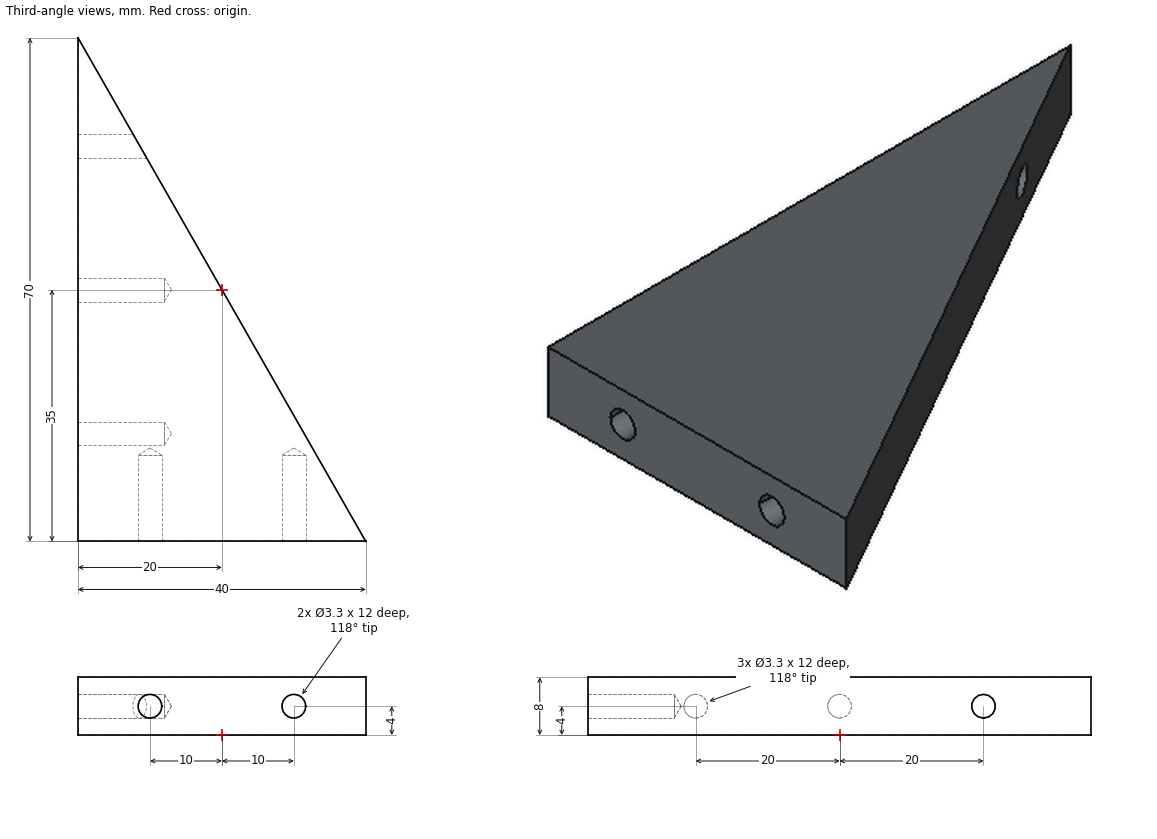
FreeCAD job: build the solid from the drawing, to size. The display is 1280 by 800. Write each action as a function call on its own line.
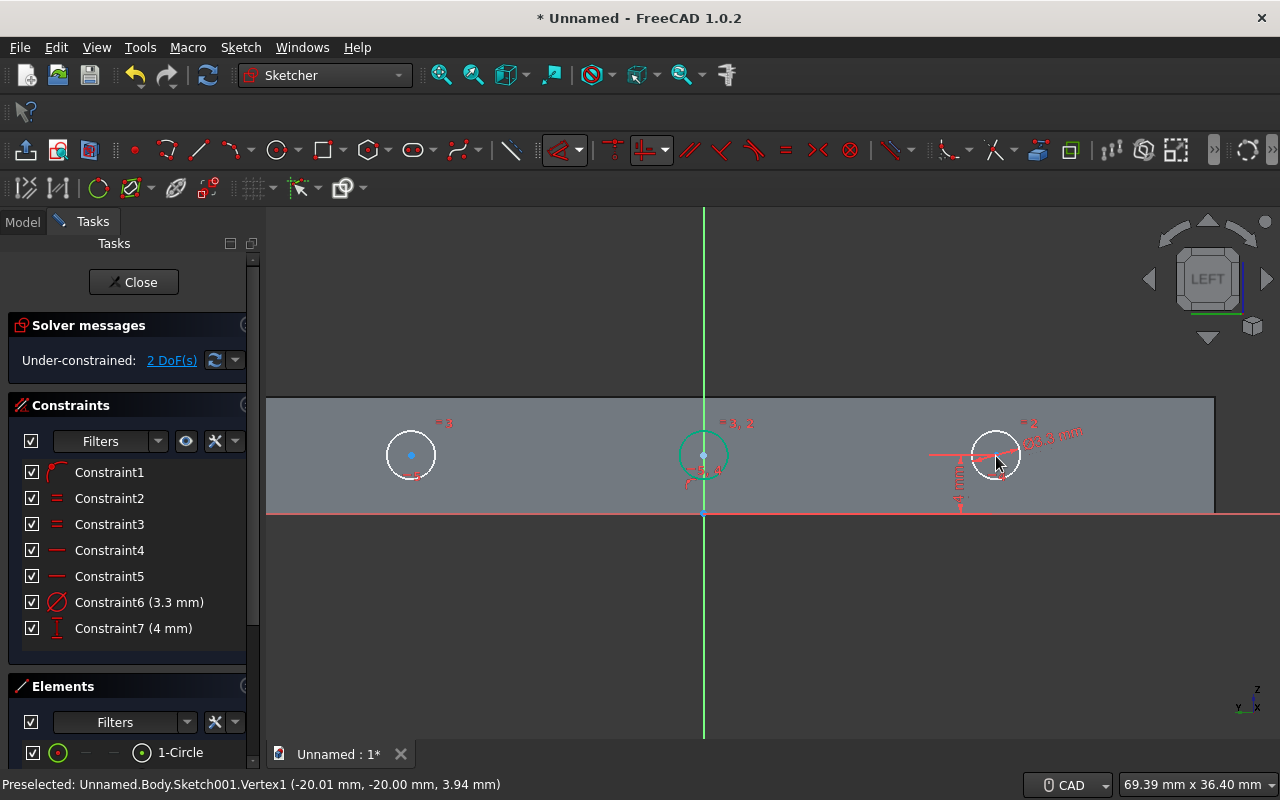
click(996, 455)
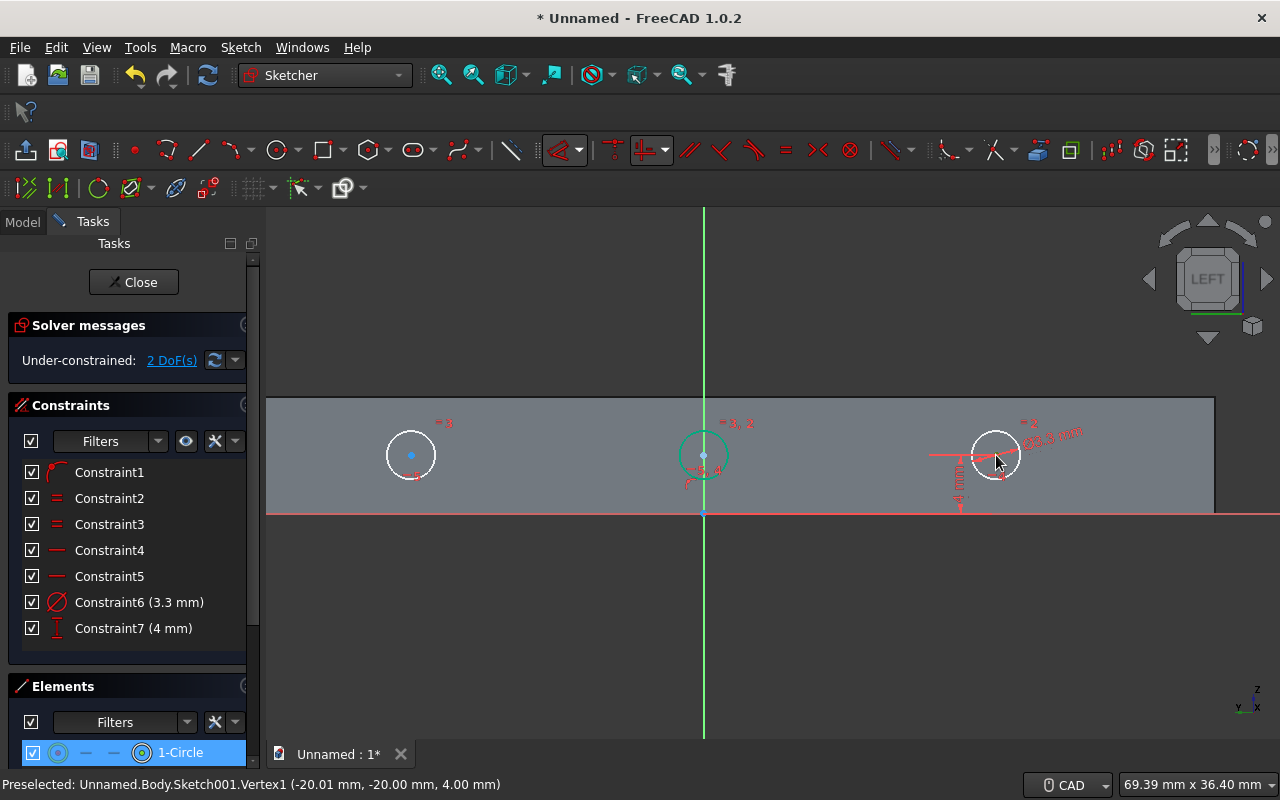
click(582, 150)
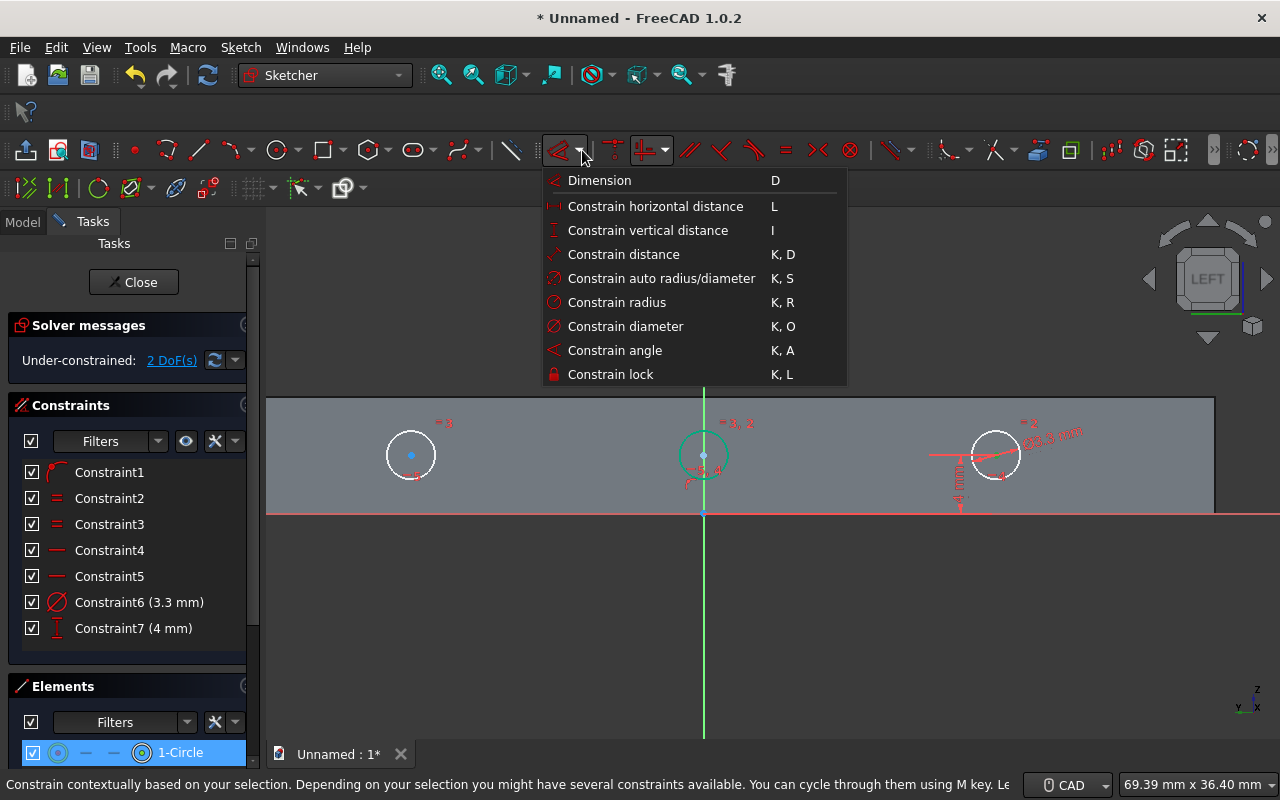
click(695, 206)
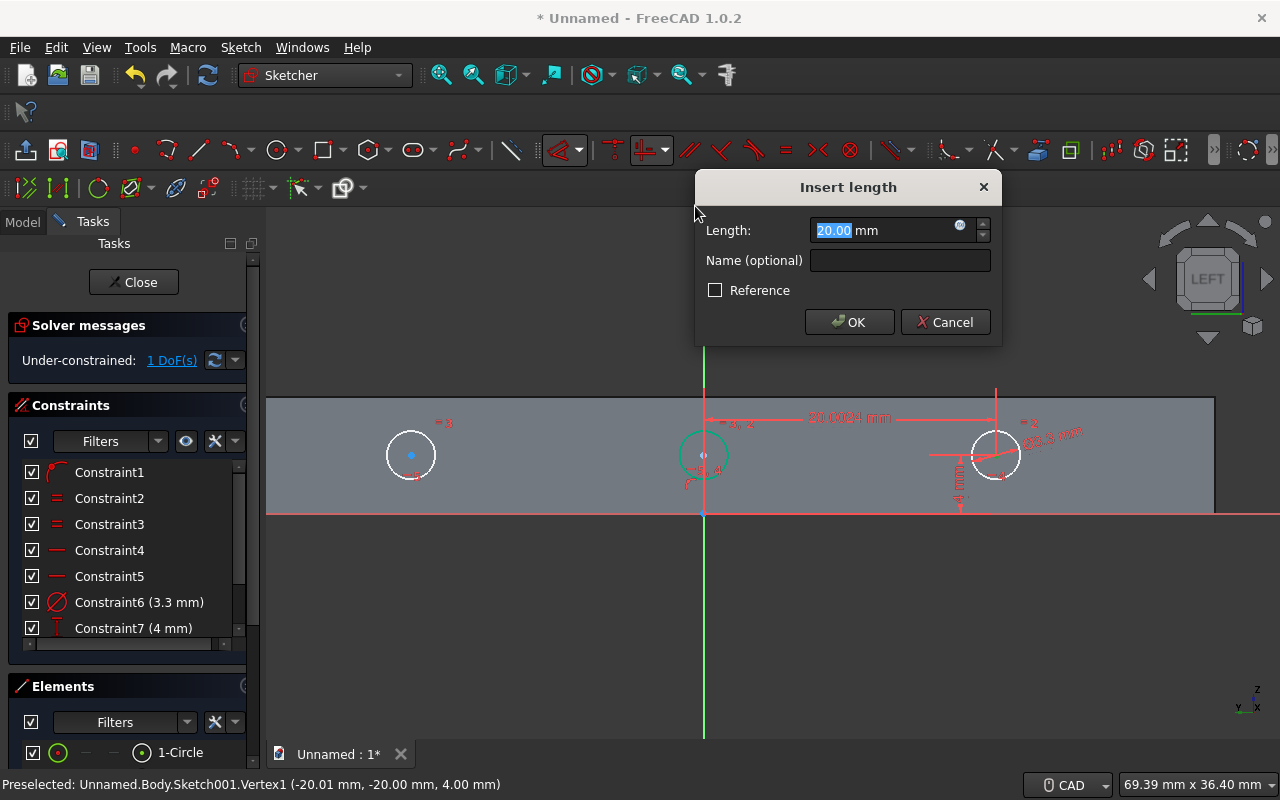
text(20)
key(Return)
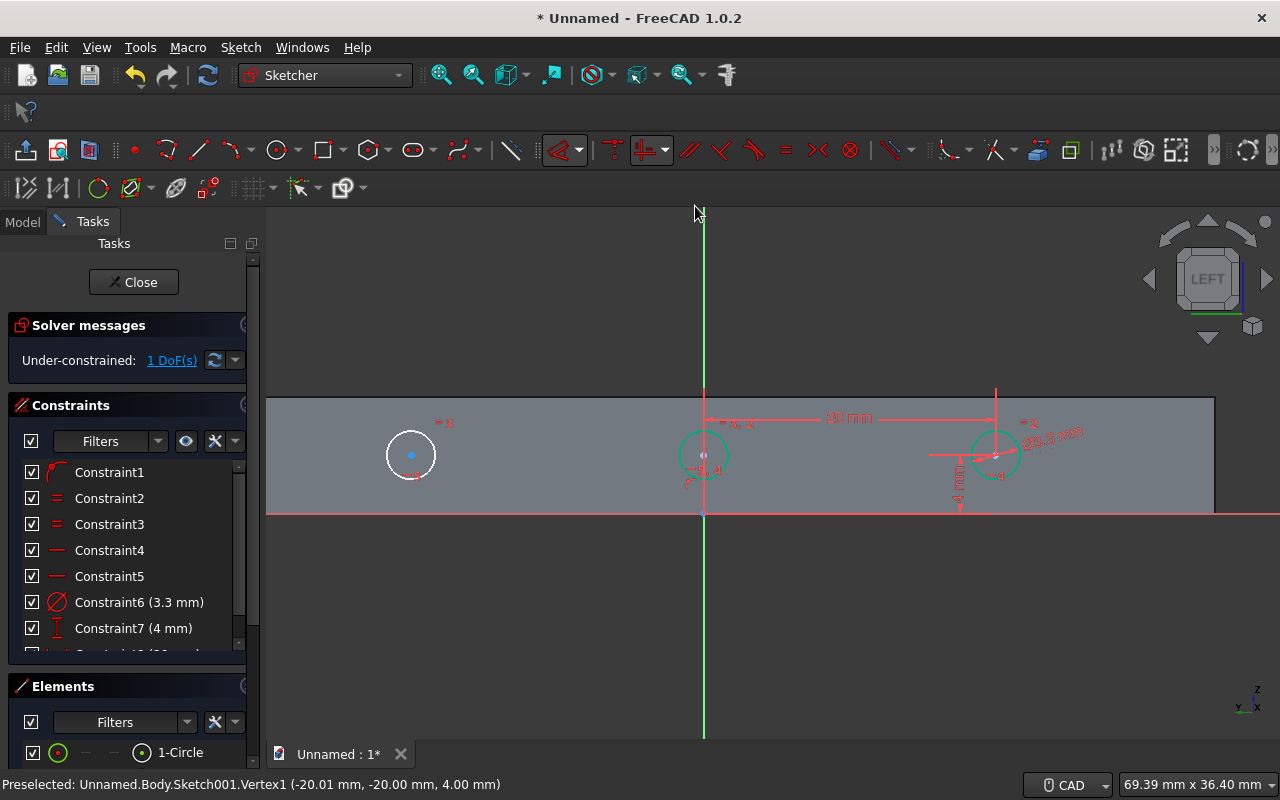
click(411, 455)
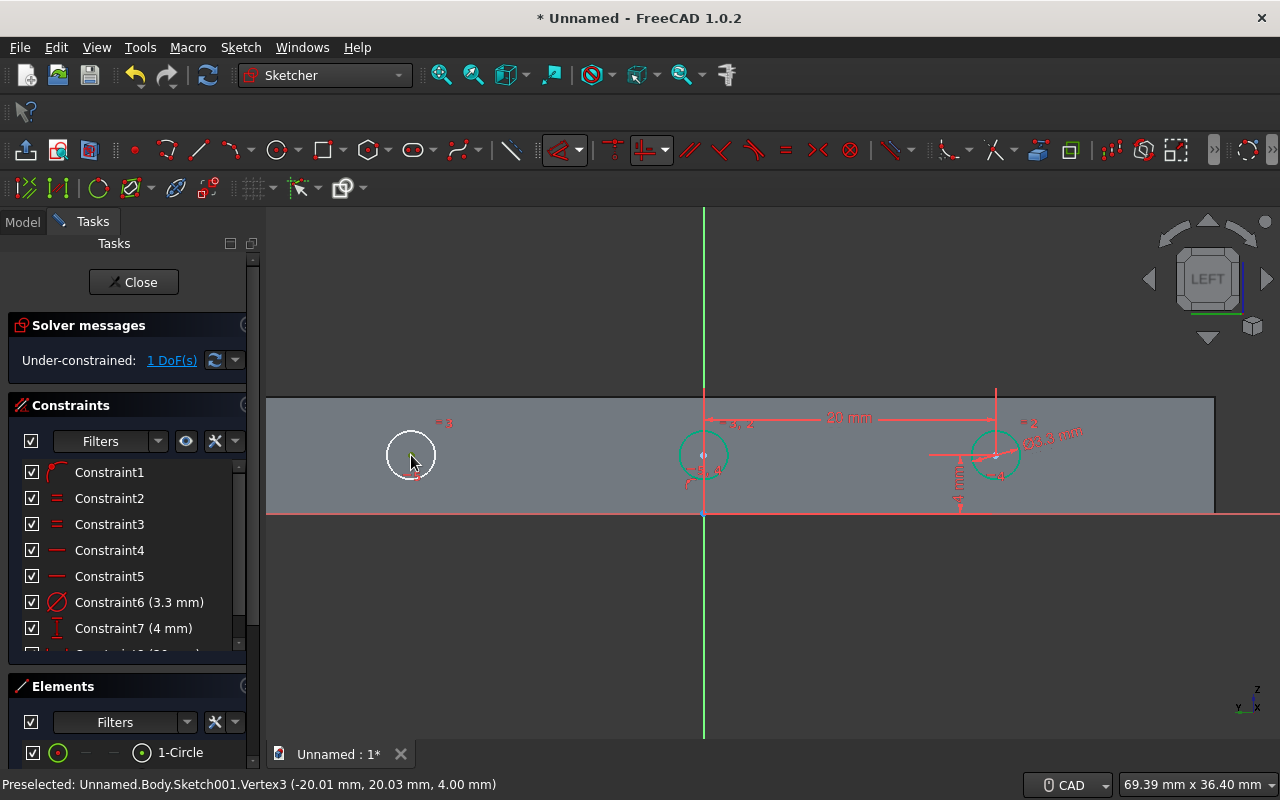
key(l)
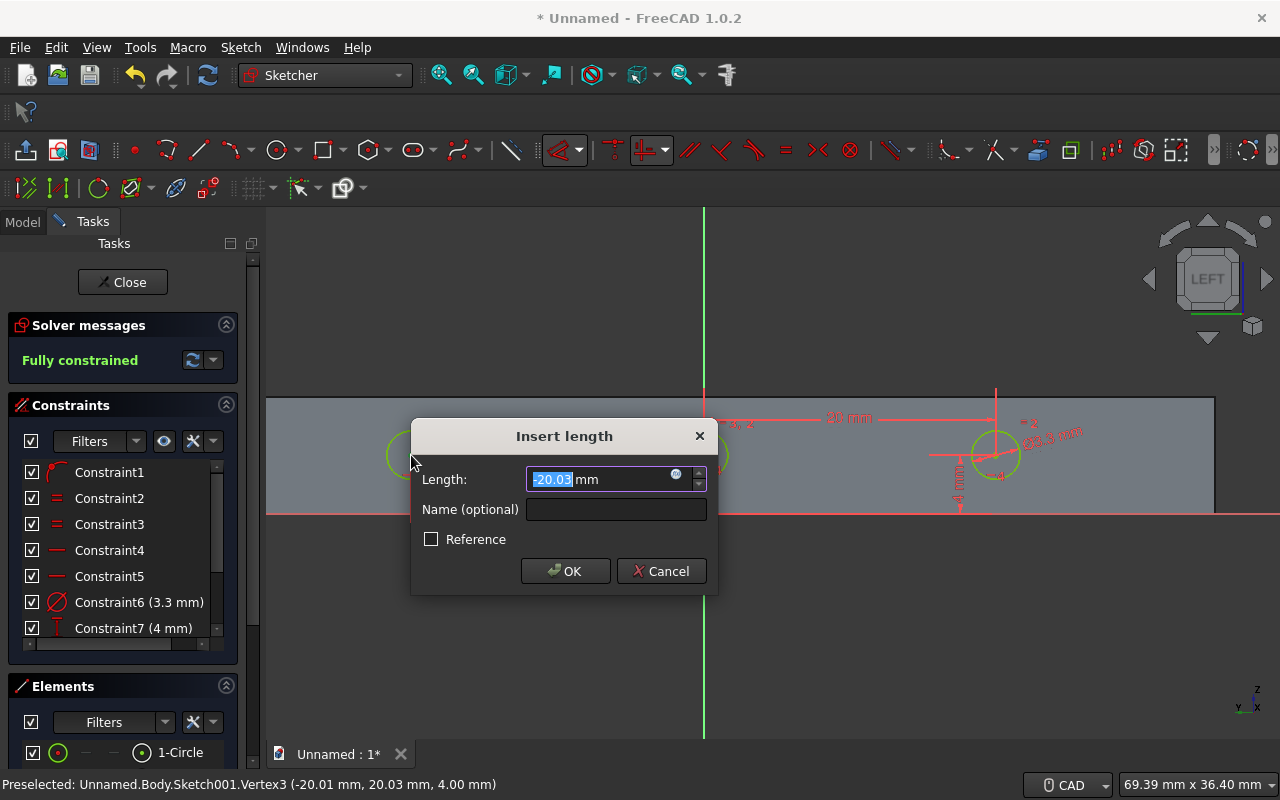
text(-20)
key(Return)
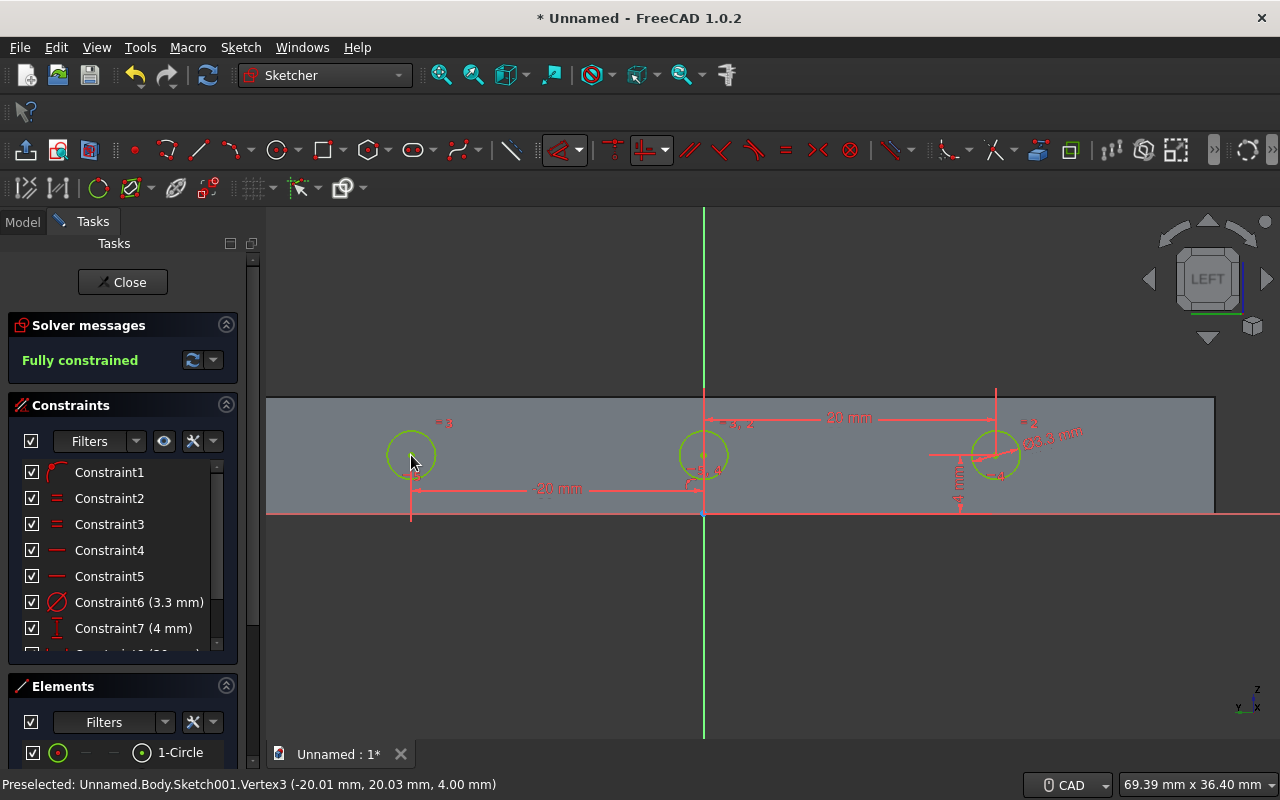
click(123, 282)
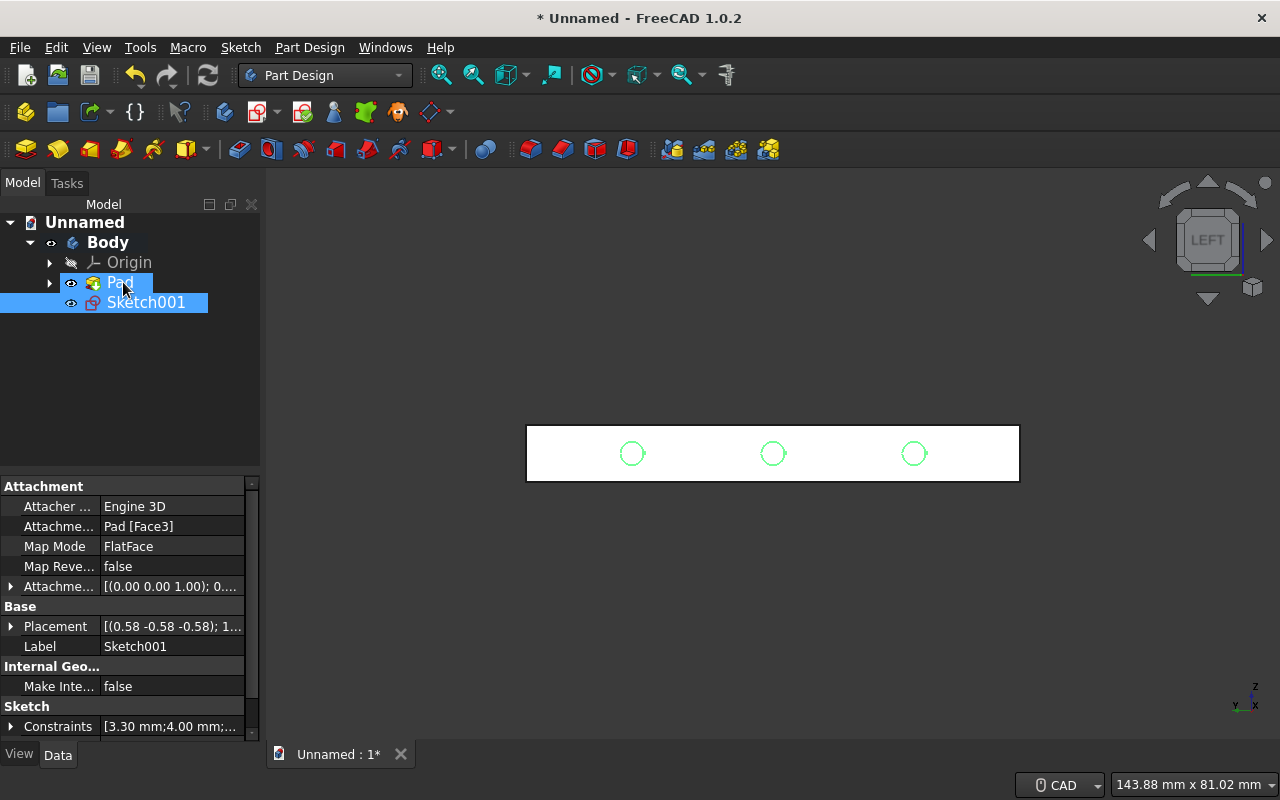
click(272, 150)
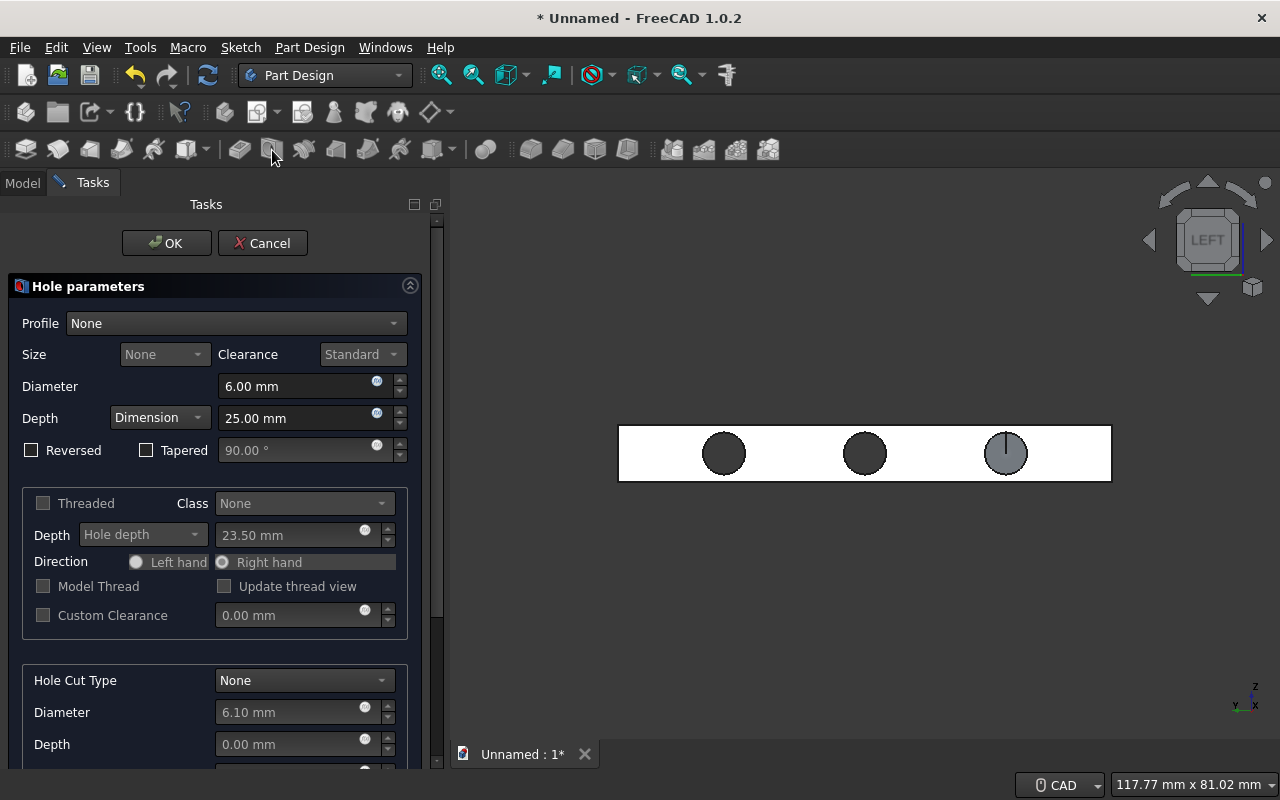
triple_click(305, 386)